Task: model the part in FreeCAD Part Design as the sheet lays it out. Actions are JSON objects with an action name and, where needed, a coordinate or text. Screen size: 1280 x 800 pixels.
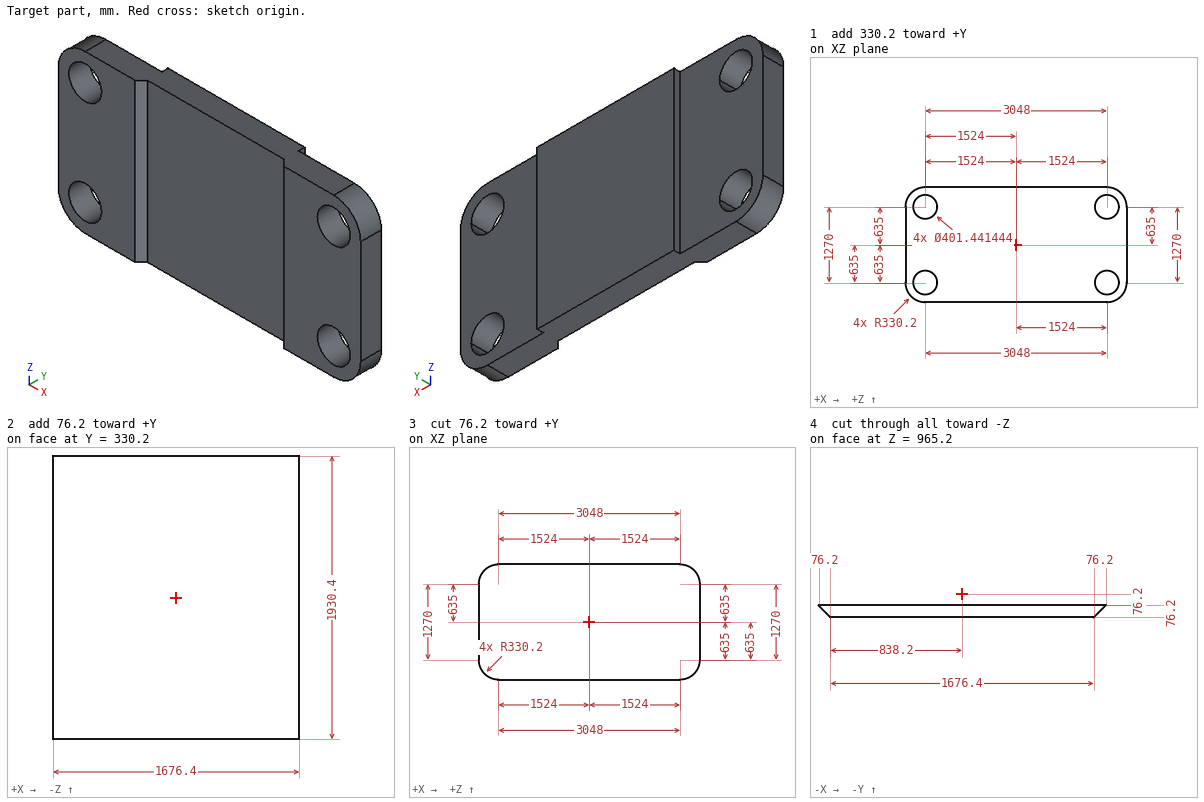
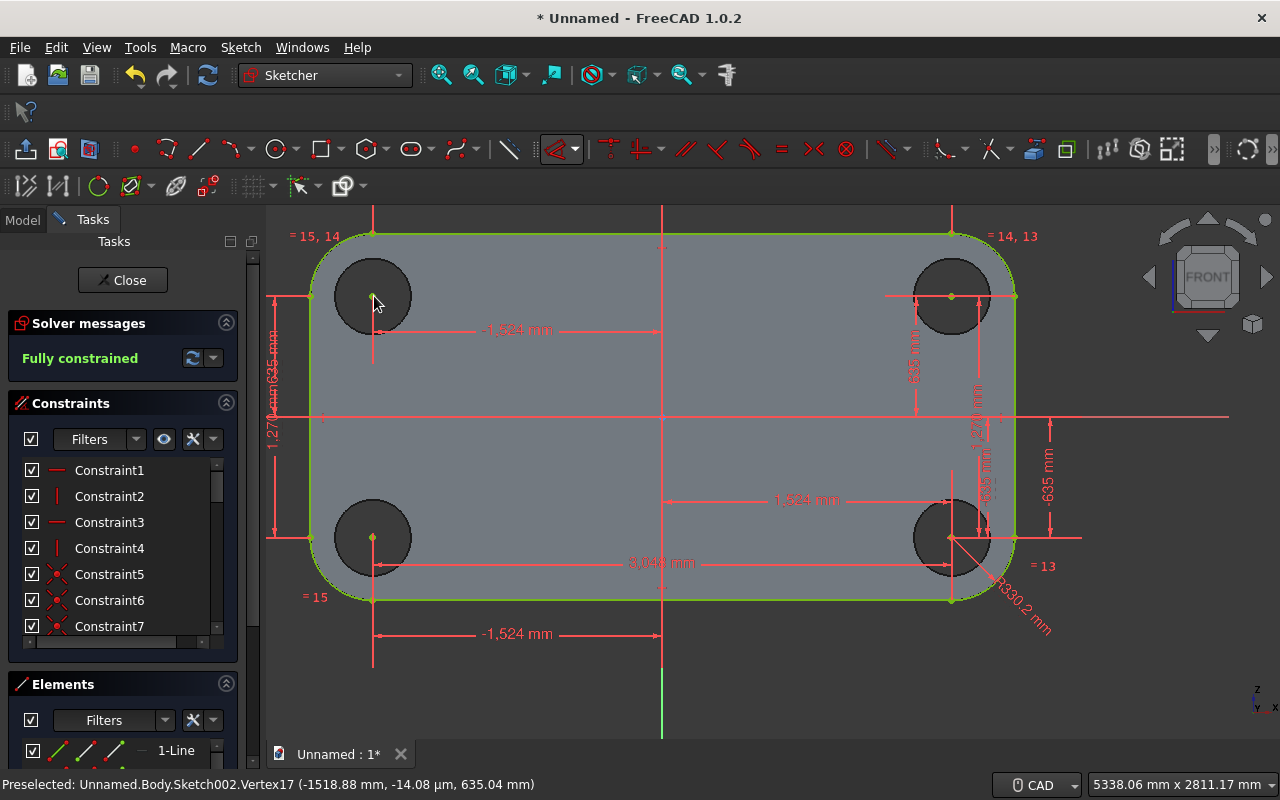
{"action": "left_click", "coordinate": [123, 280]}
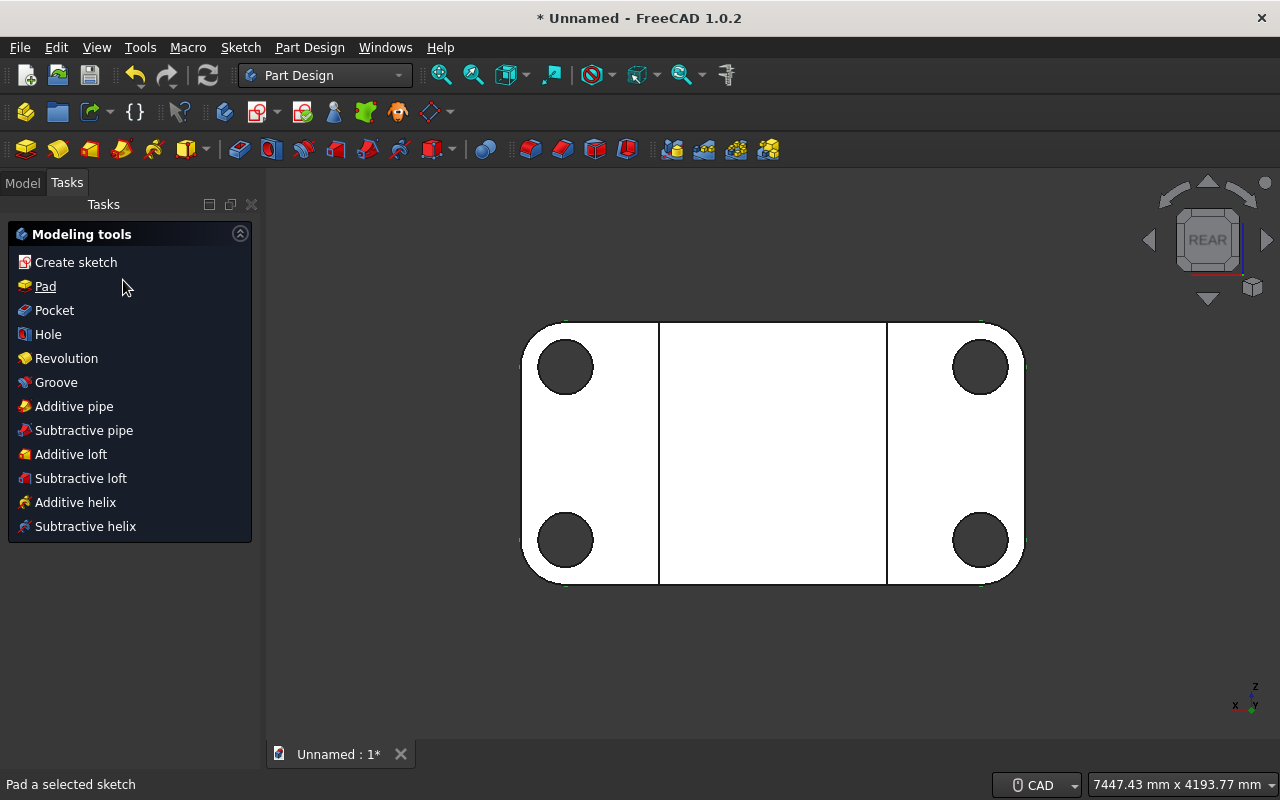
{"action": "left_click", "coordinate": [240, 150]}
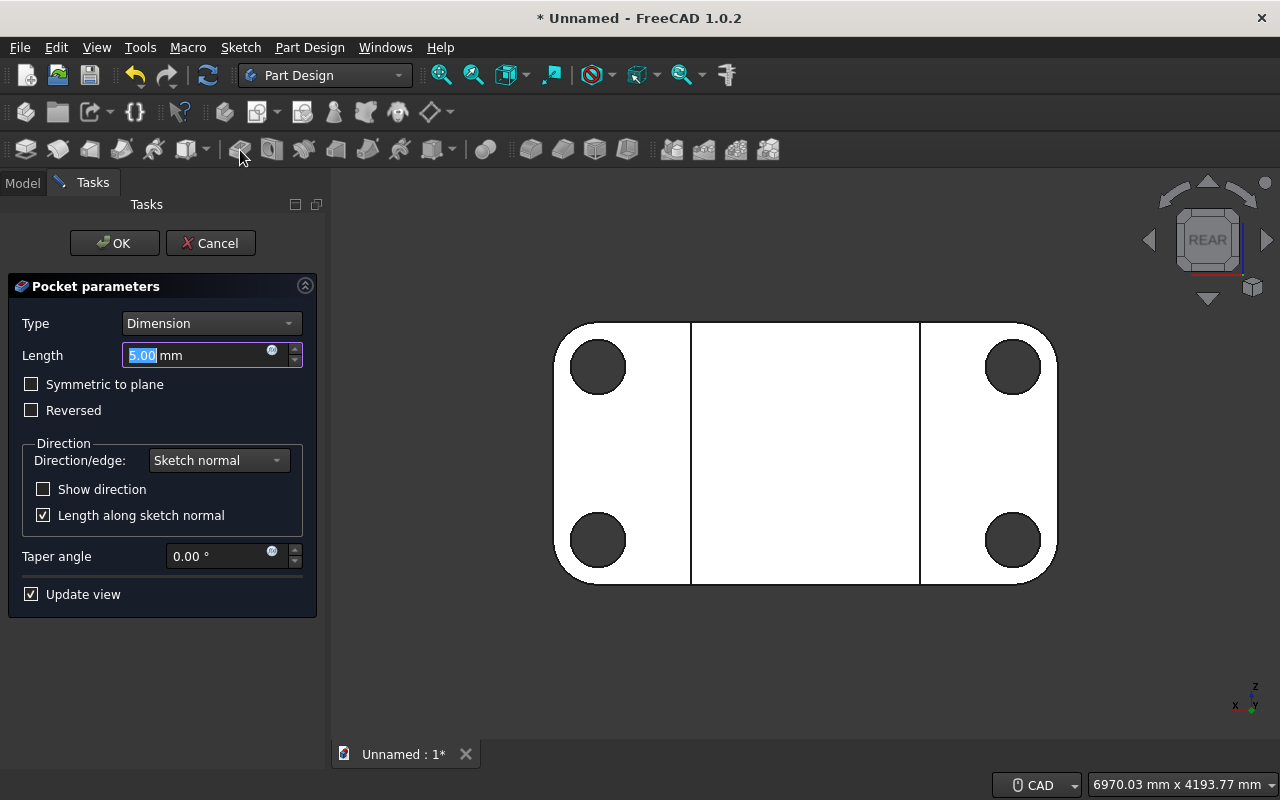
{"action": "type", "text": "76.2"}
{"action": "key", "text": "Tab"}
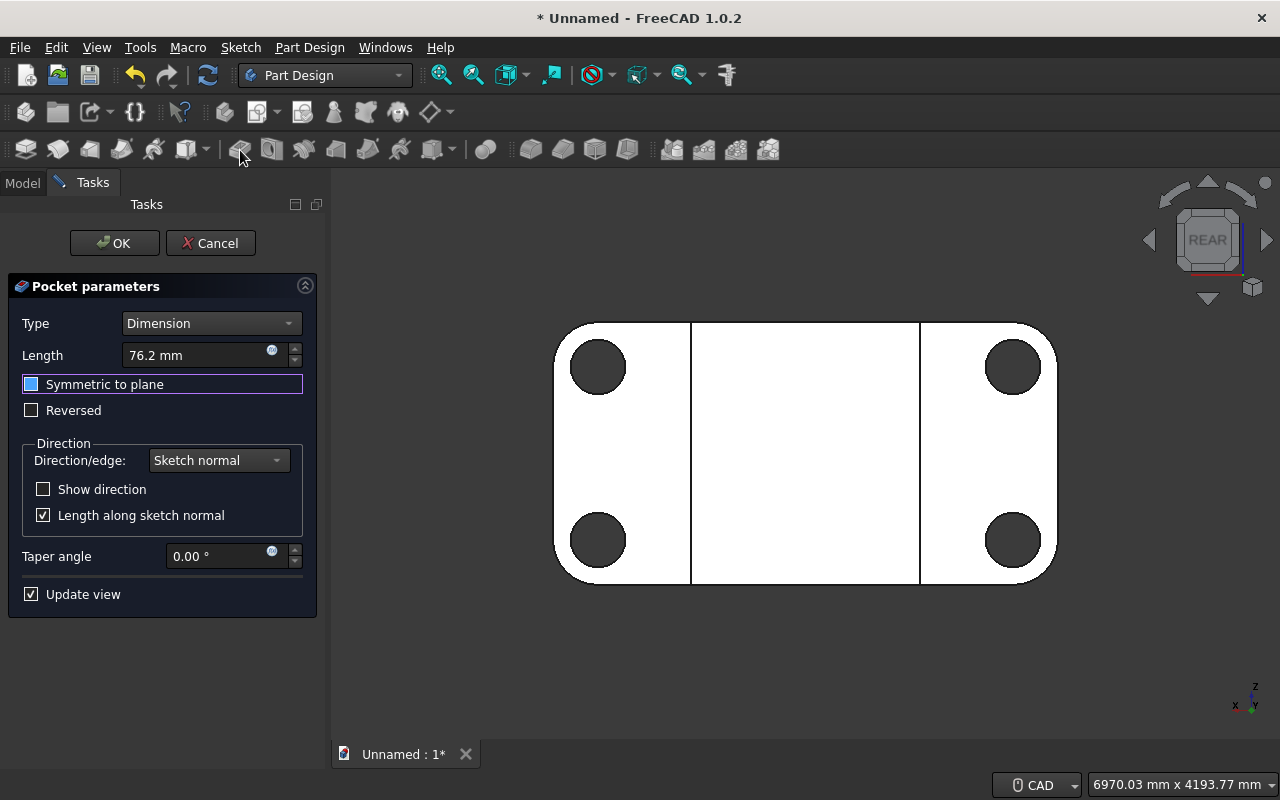
{"action": "left_click", "coordinate": [115, 243]}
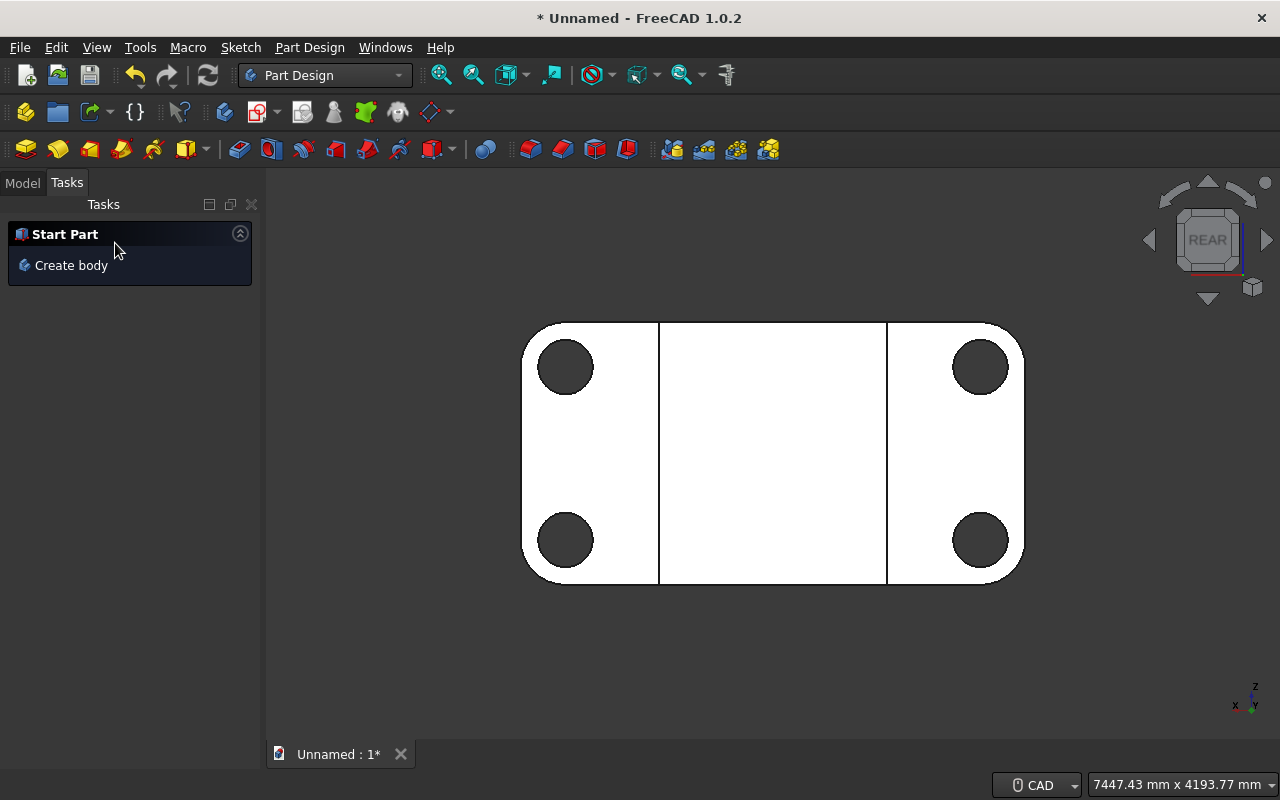
{"action": "key", "text": "0"}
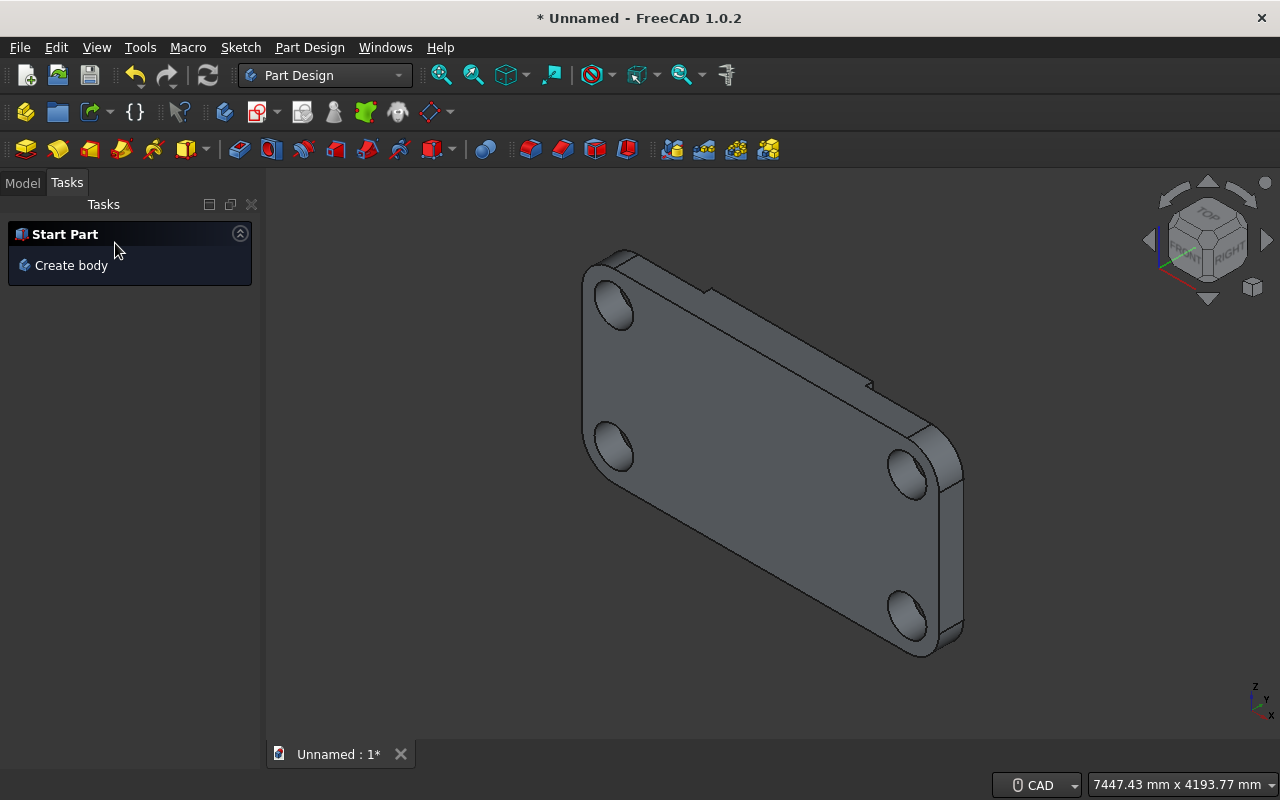
{"action": "left_click", "coordinate": [818, 367]}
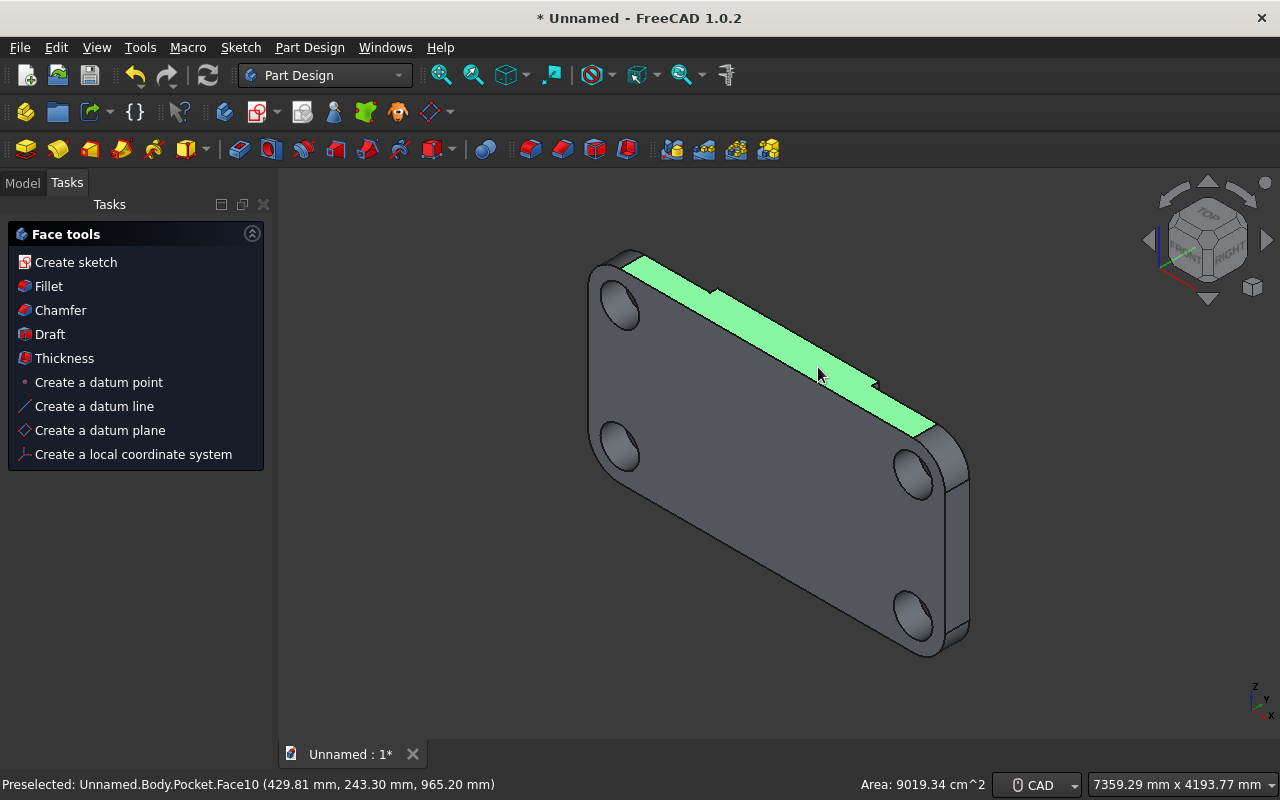
{"action": "left_click", "coordinate": [258, 112]}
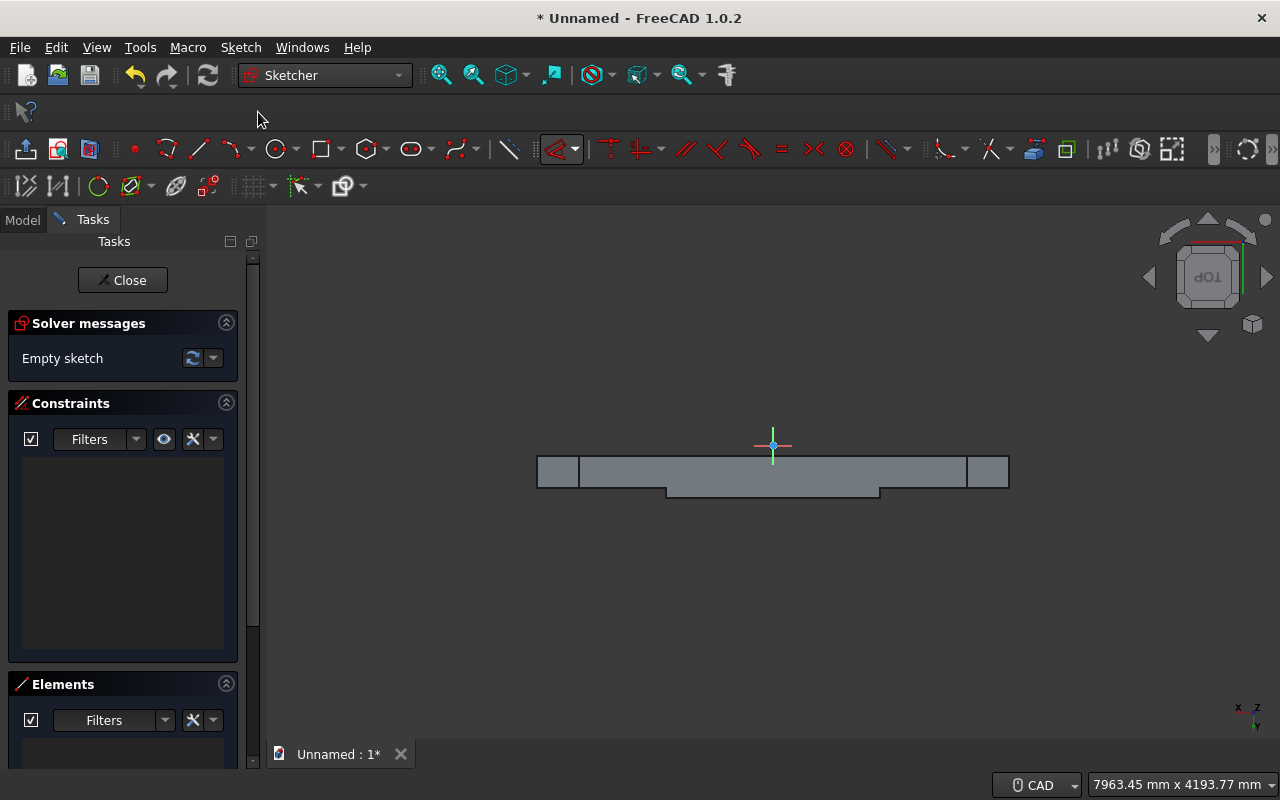
{"action": "scroll", "coordinate": [813, 446], "scroll_direction": "up", "scroll_amount": 5}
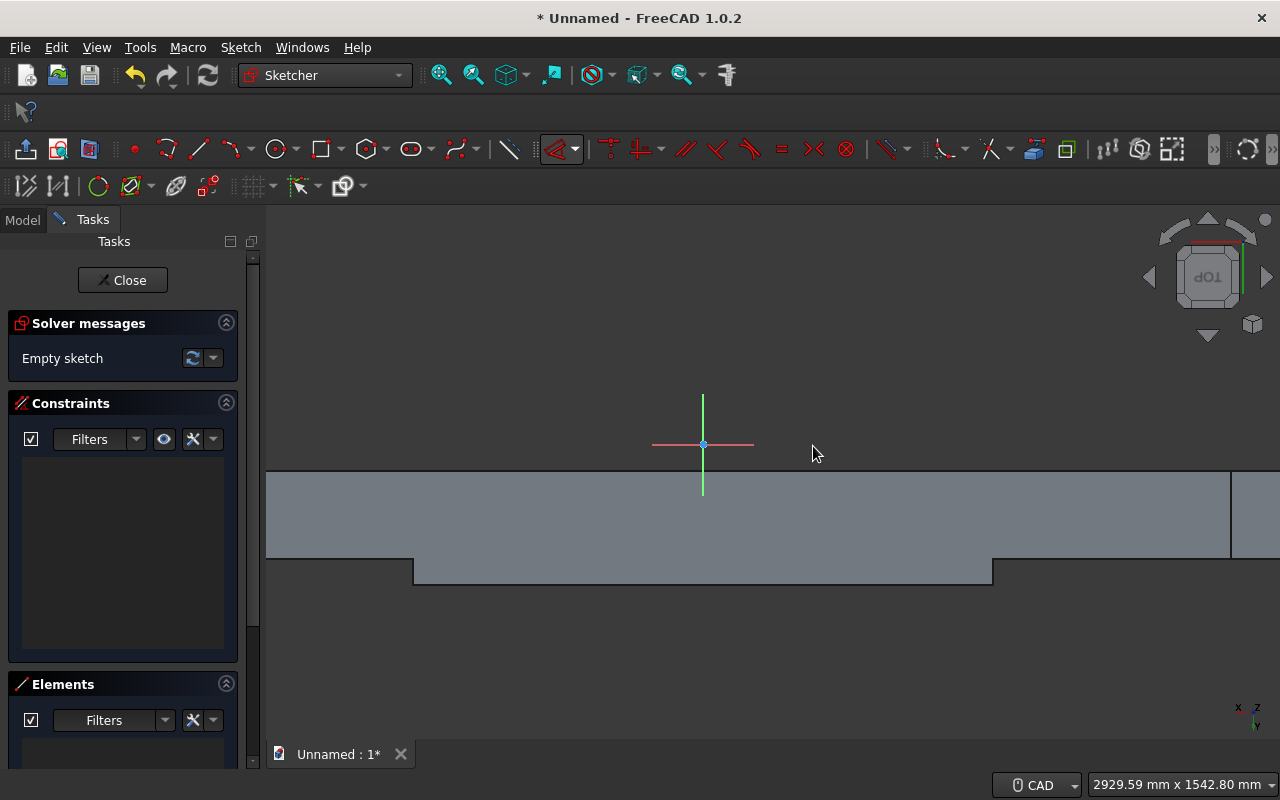
{"action": "key", "text": "g m"}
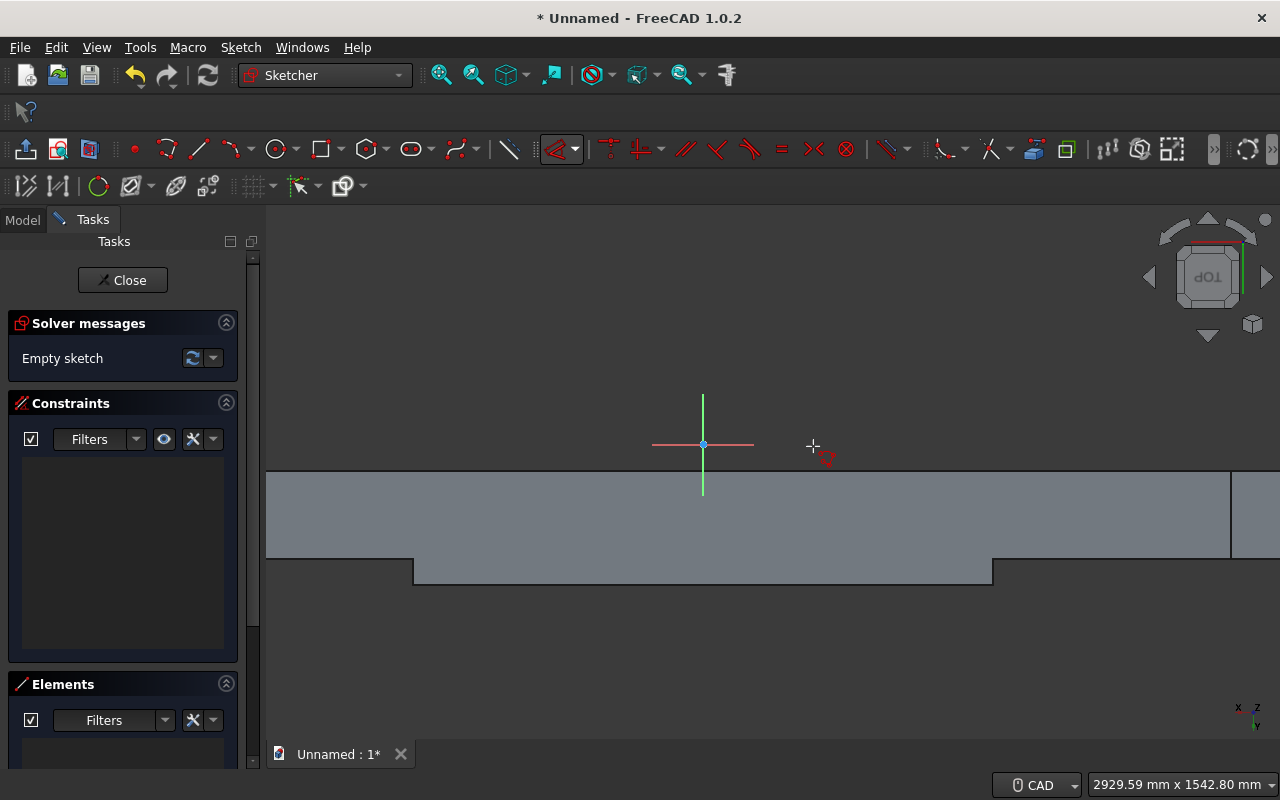
{"action": "left_click", "coordinate": [413, 497]}
{"action": "left_click", "coordinate": [993, 497]}
{"action": "left_click", "coordinate": [1020, 471]}
{"action": "left_click", "coordinate": [387, 471]}
{"action": "left_click", "coordinate": [413, 498]}
{"action": "key", "text": "Escape"}
{"action": "key", "text": "Escape"}